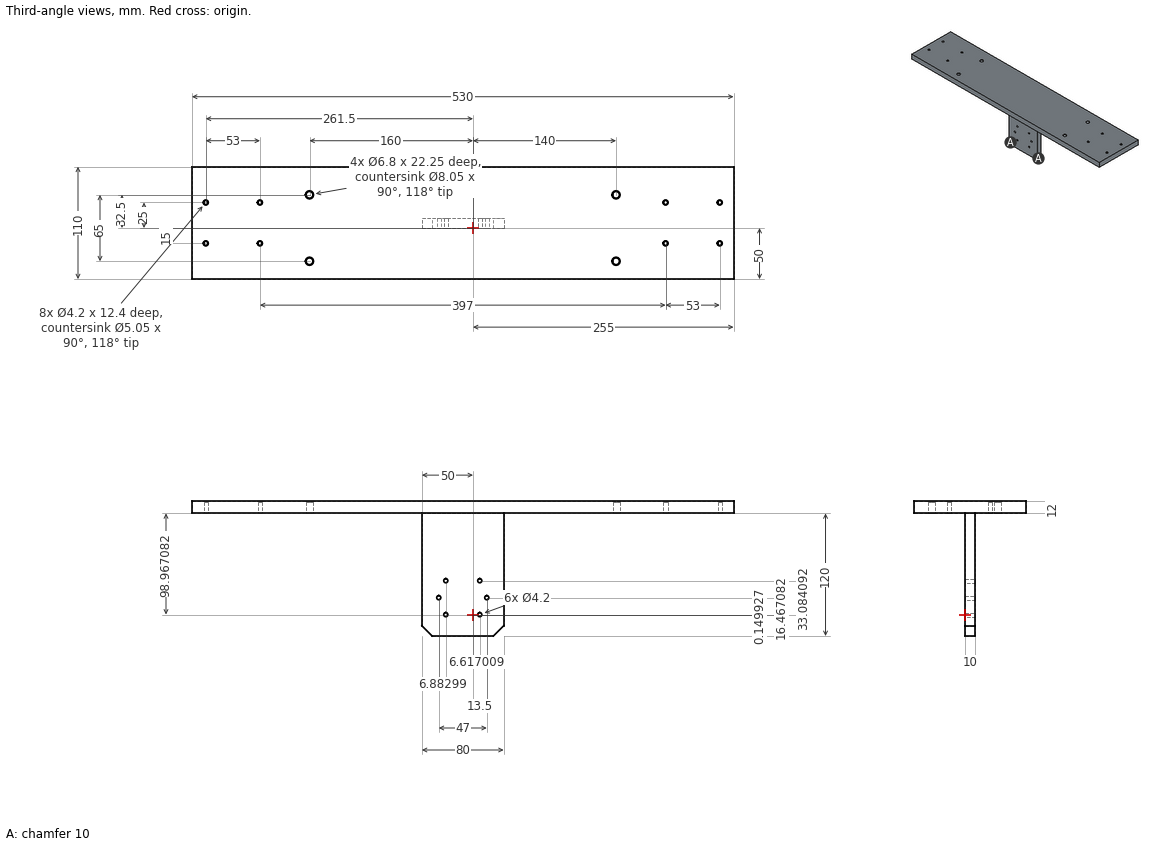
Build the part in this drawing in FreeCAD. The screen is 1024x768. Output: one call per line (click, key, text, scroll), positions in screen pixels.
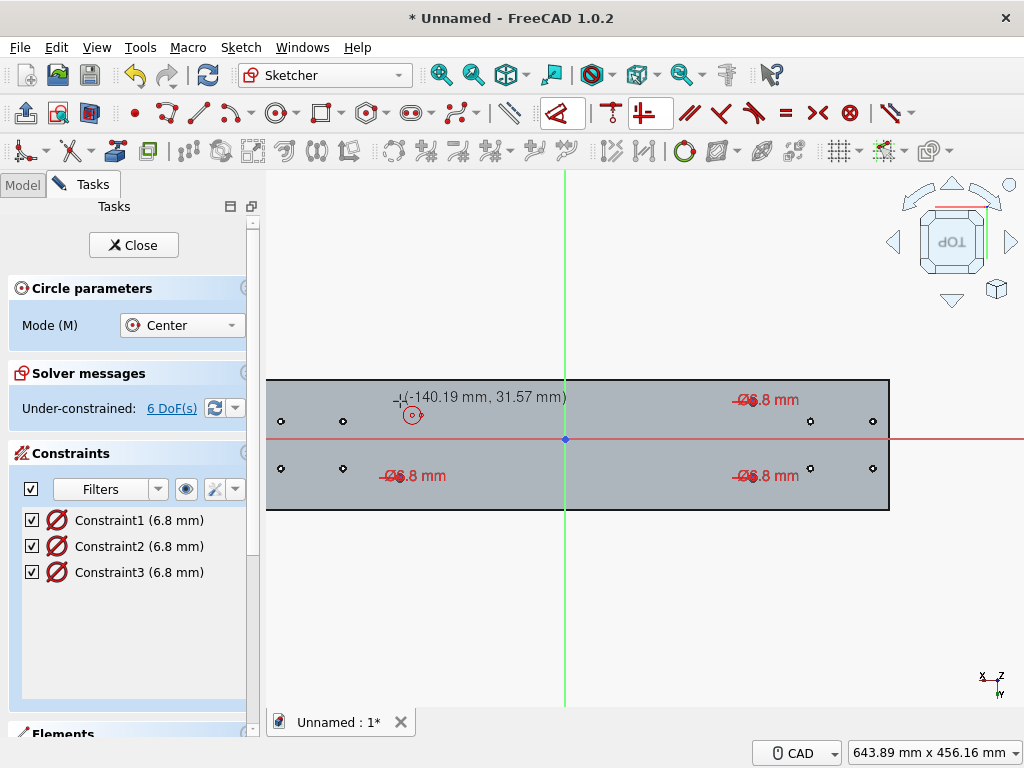
click(400, 401)
move(403, 398)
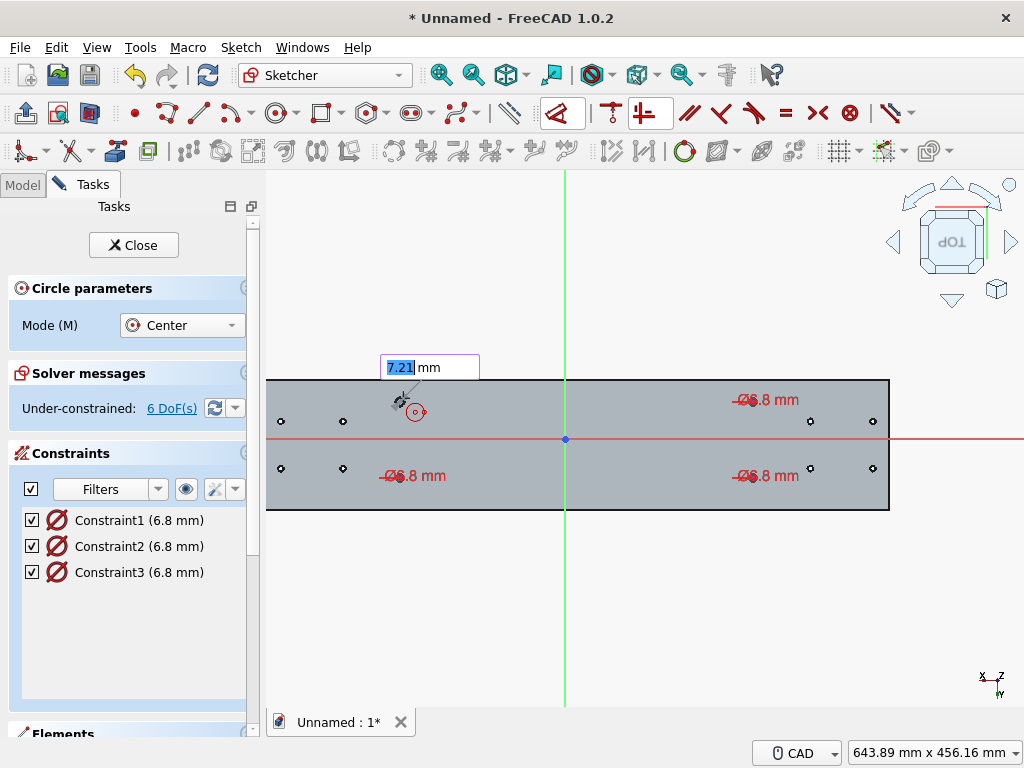
text(6.8)
key(Return)
key(Escape)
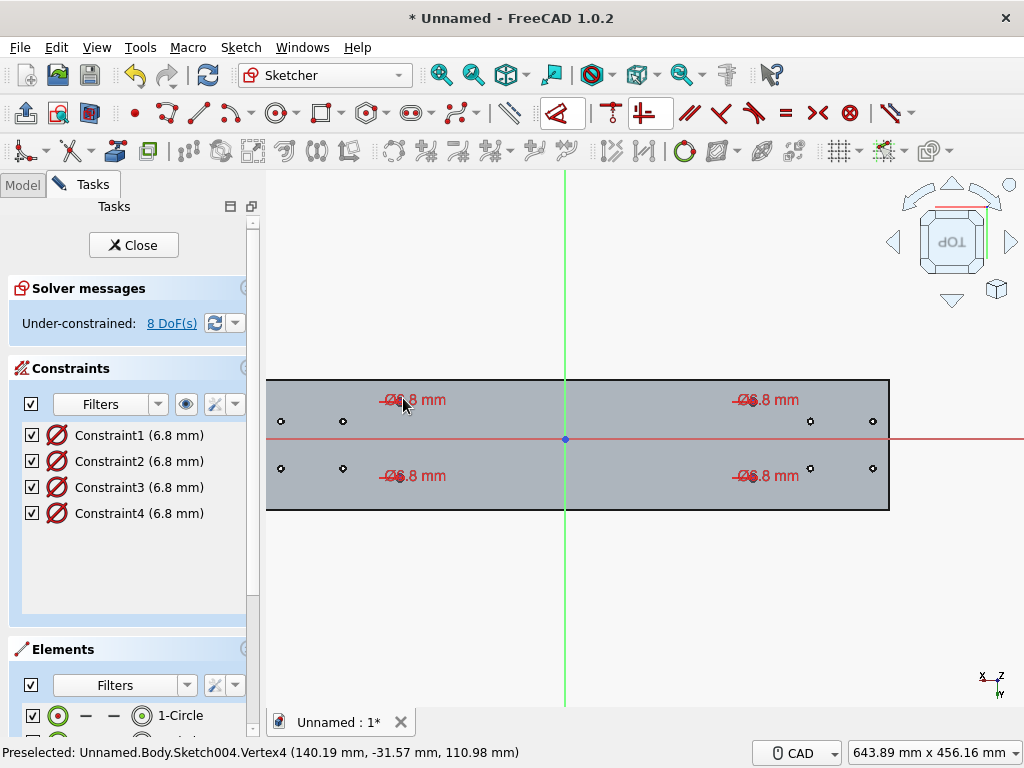
click(753, 478)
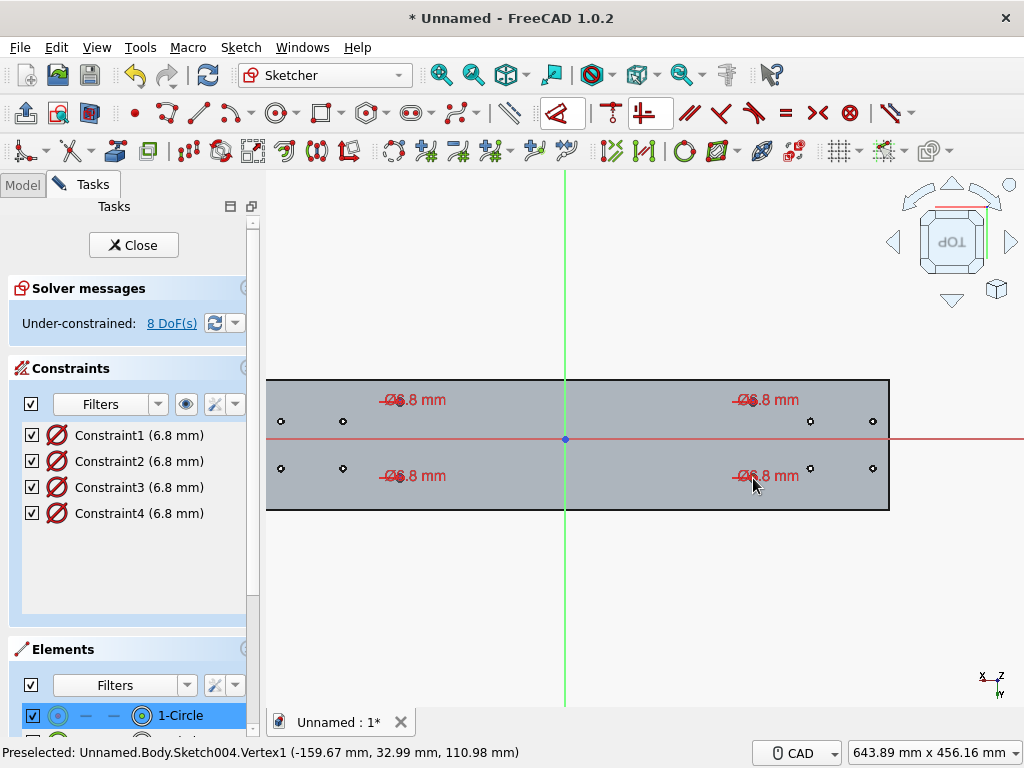
click(753, 402)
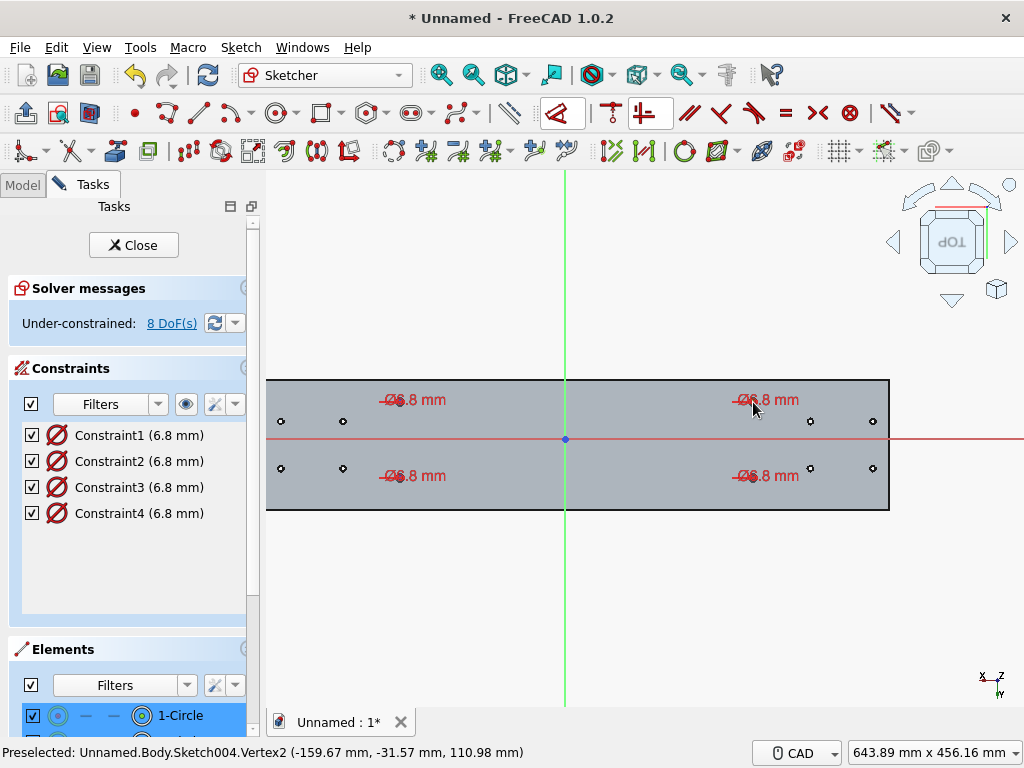
key(v)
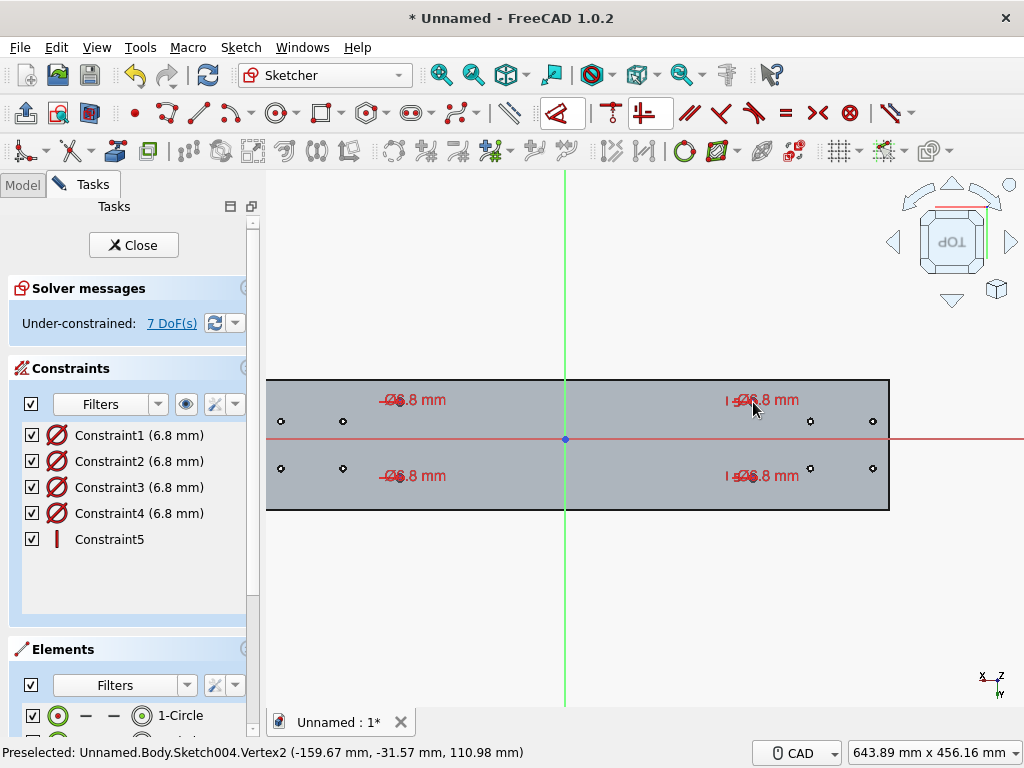
click(753, 478)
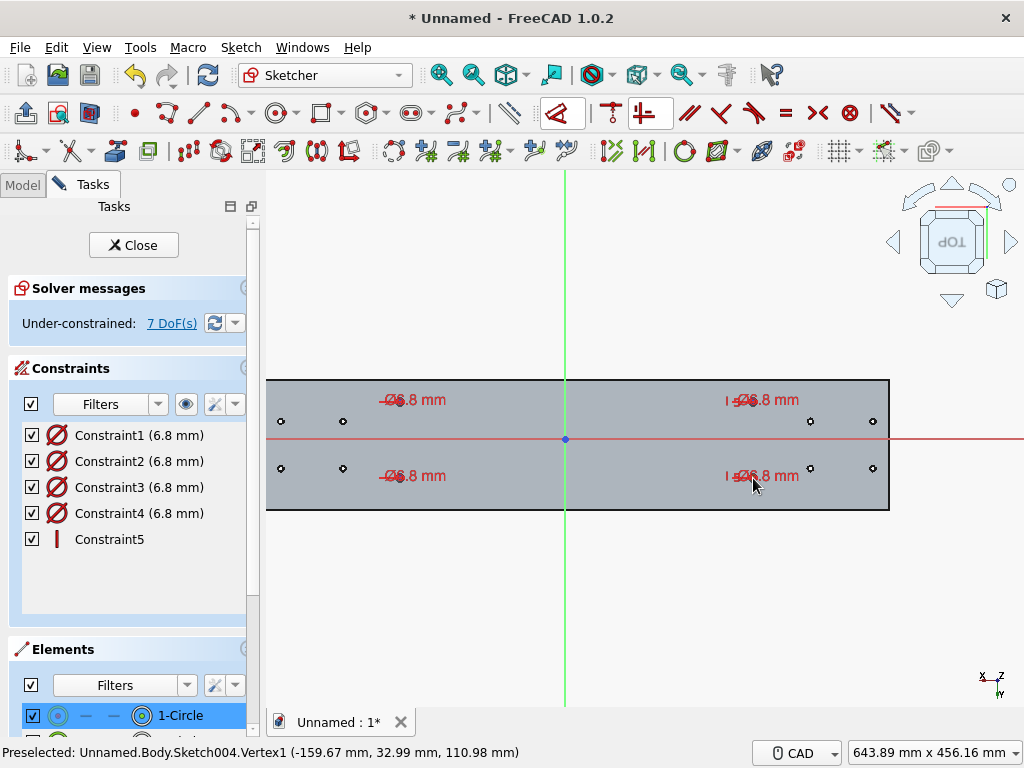
click(400, 478)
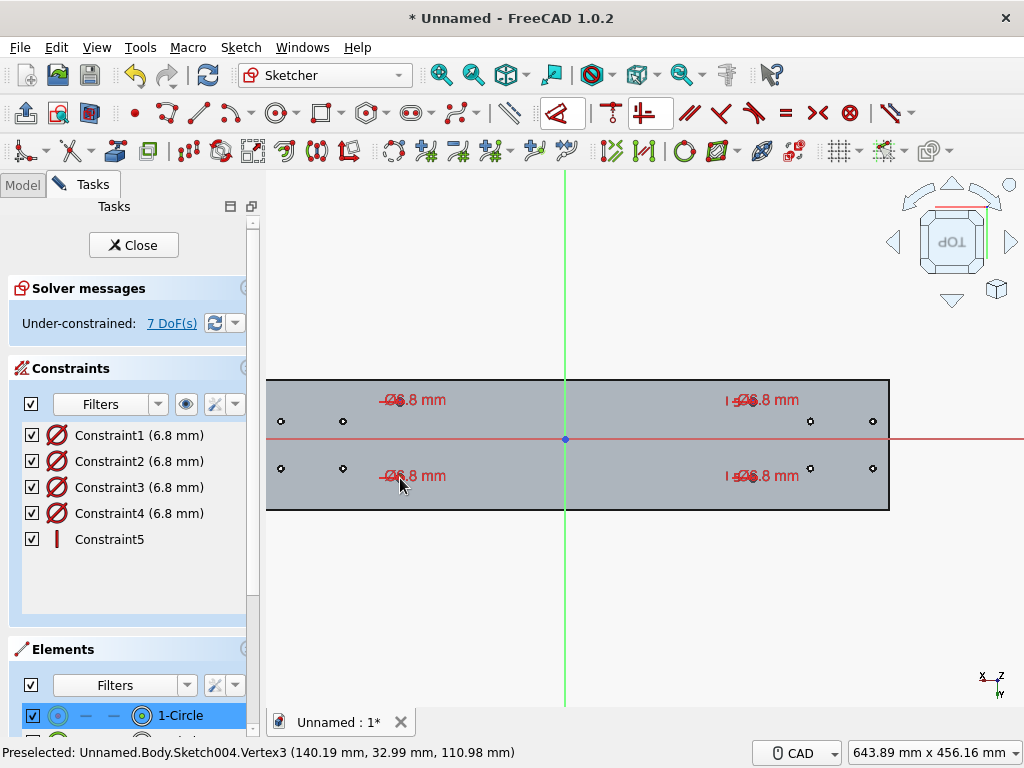
key(h)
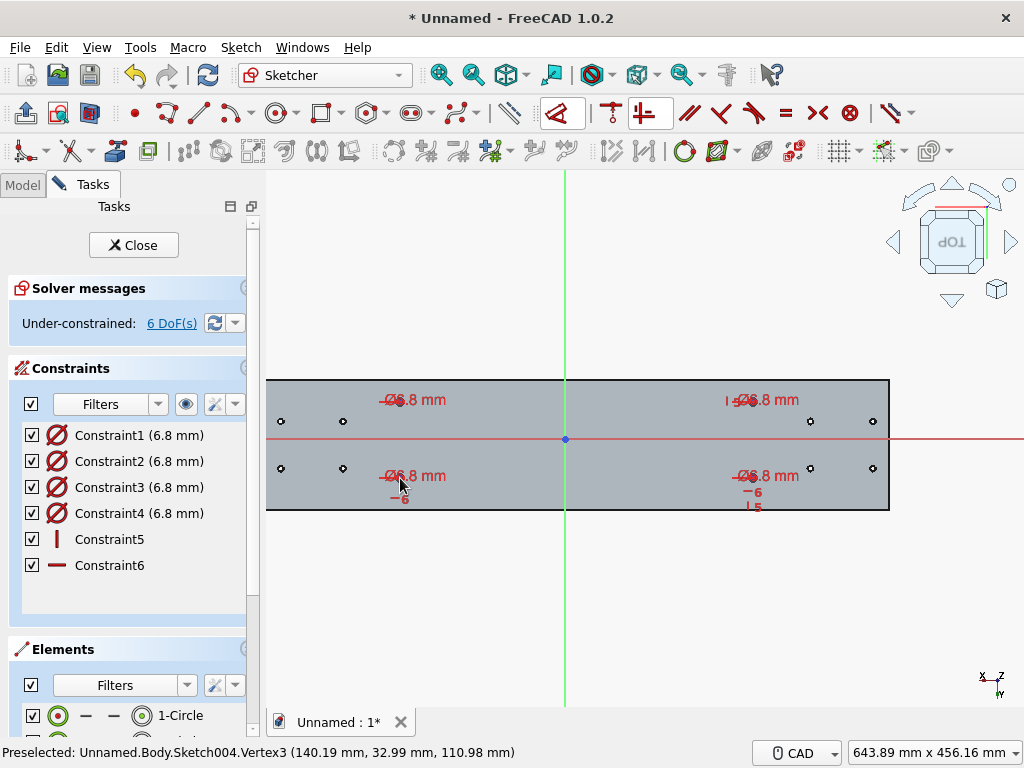
click(400, 478)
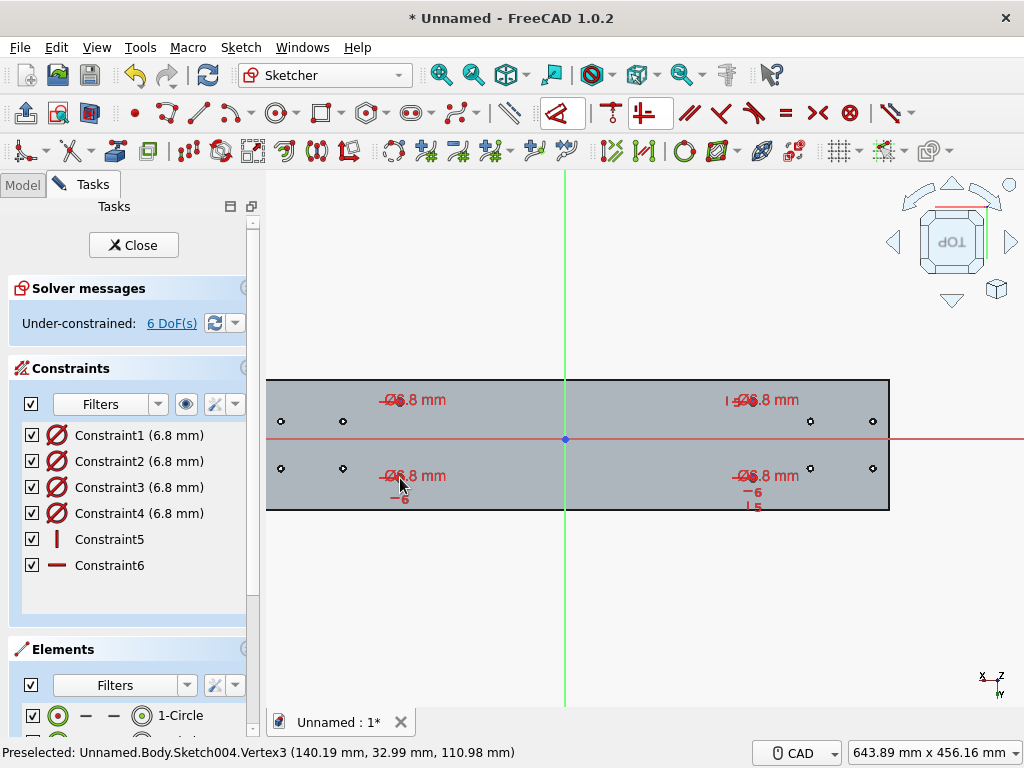
click(400, 402)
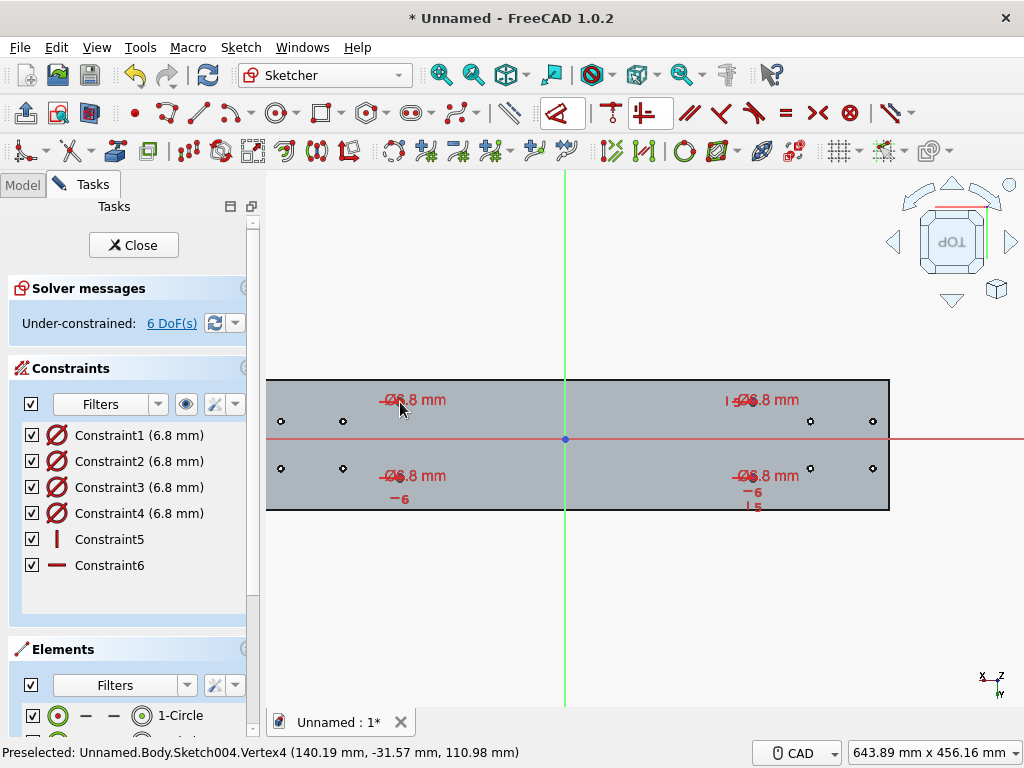
key(v)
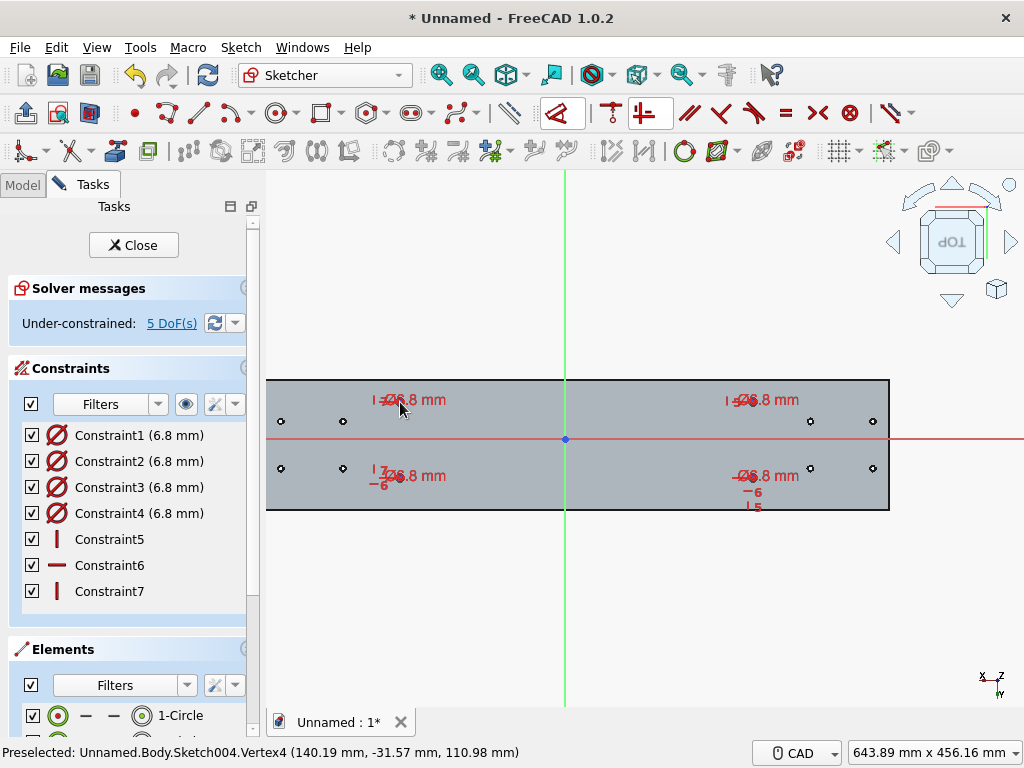
click(753, 402)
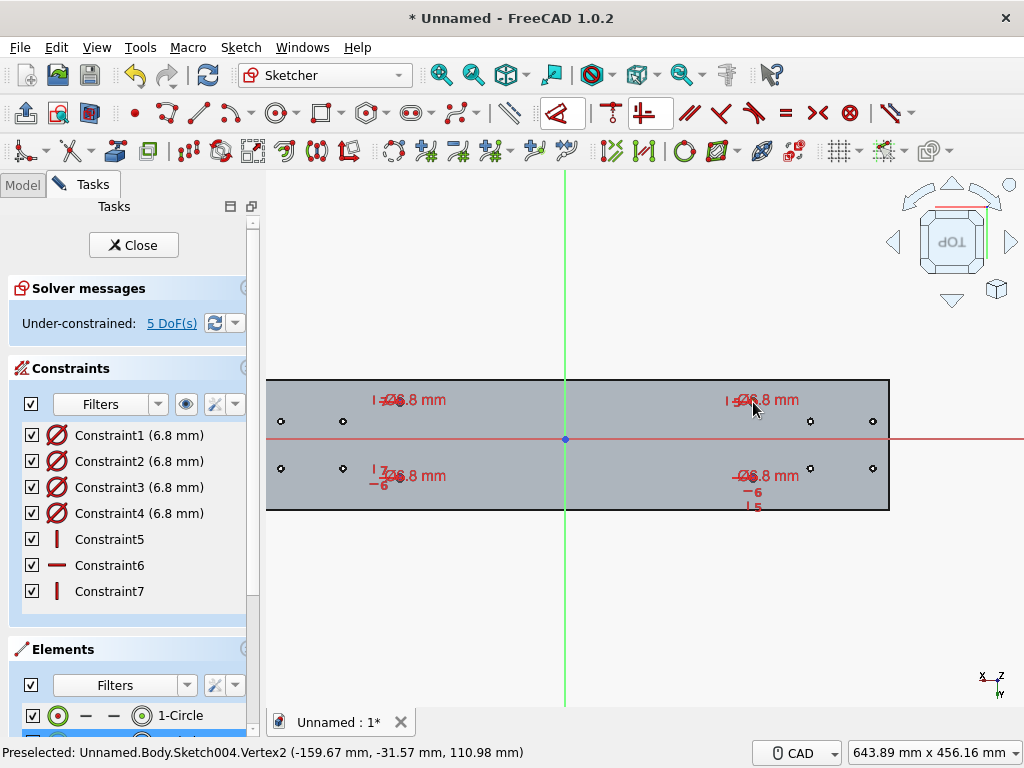
click(400, 402)